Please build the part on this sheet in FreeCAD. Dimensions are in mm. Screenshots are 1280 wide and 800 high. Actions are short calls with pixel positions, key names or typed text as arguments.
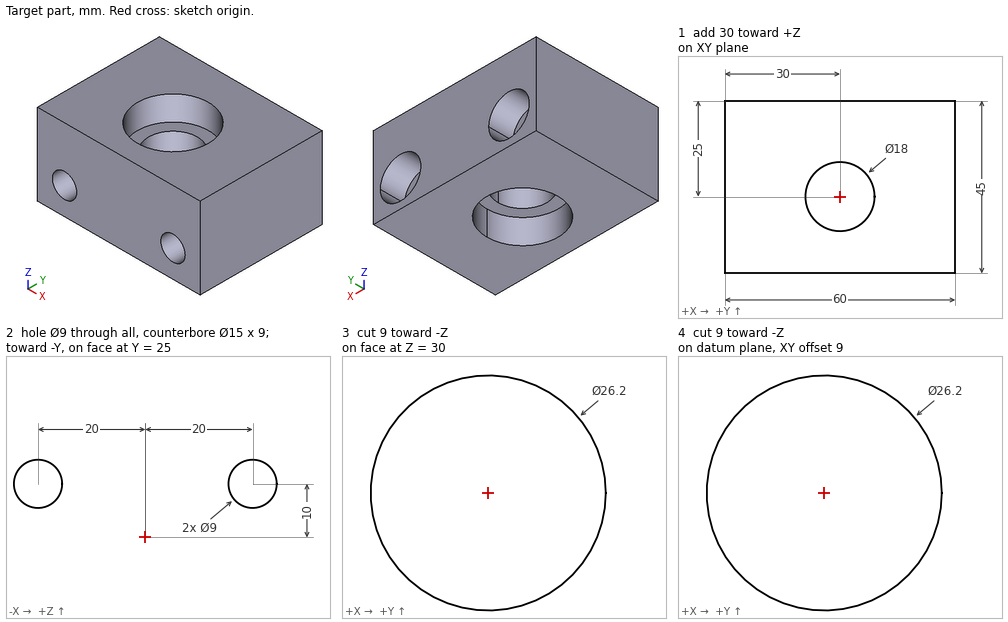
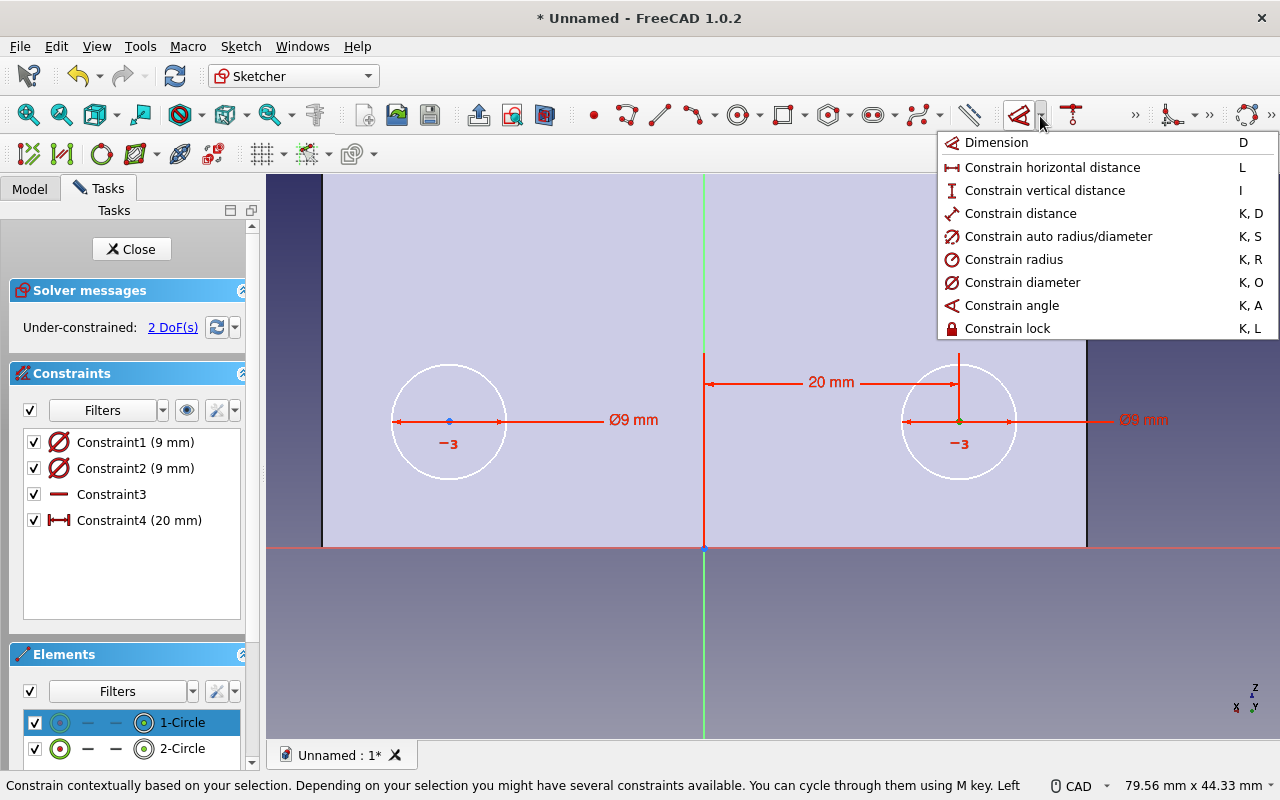
click(1108, 190)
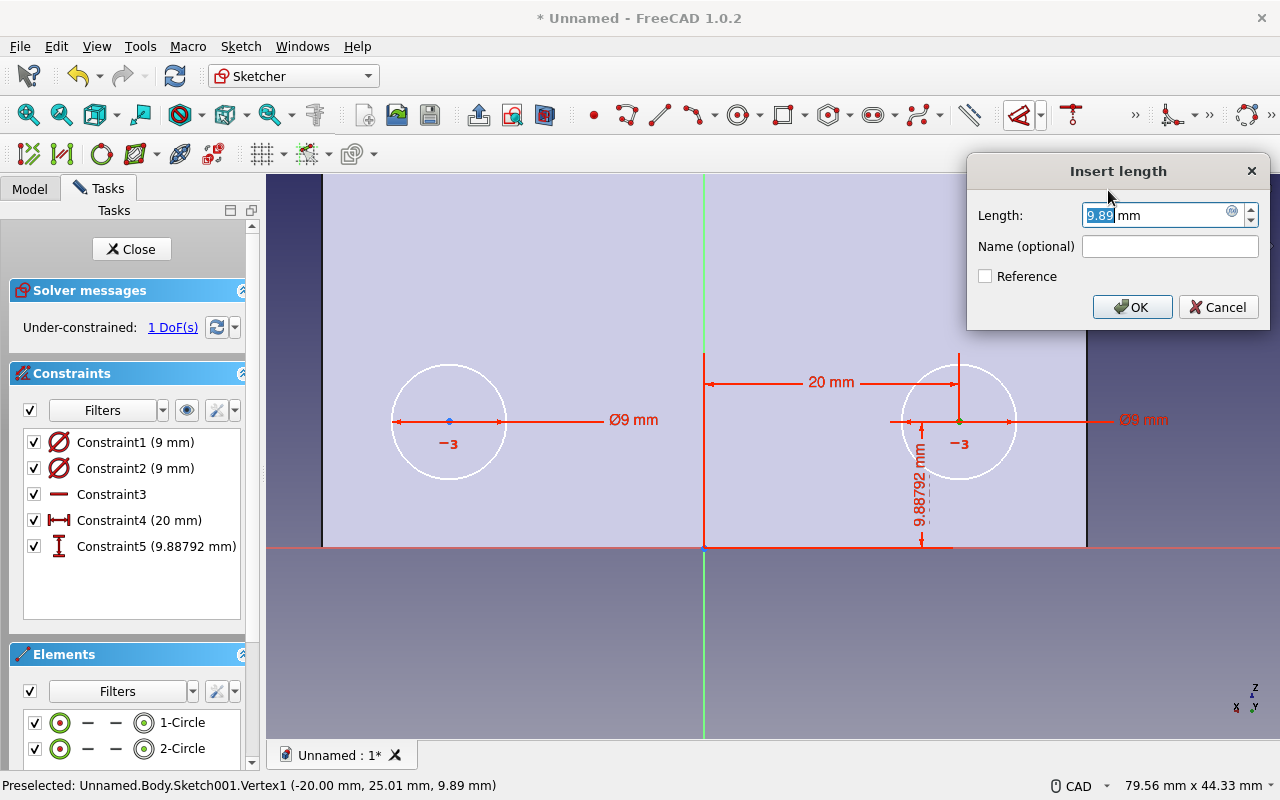
text(10)
key(Return)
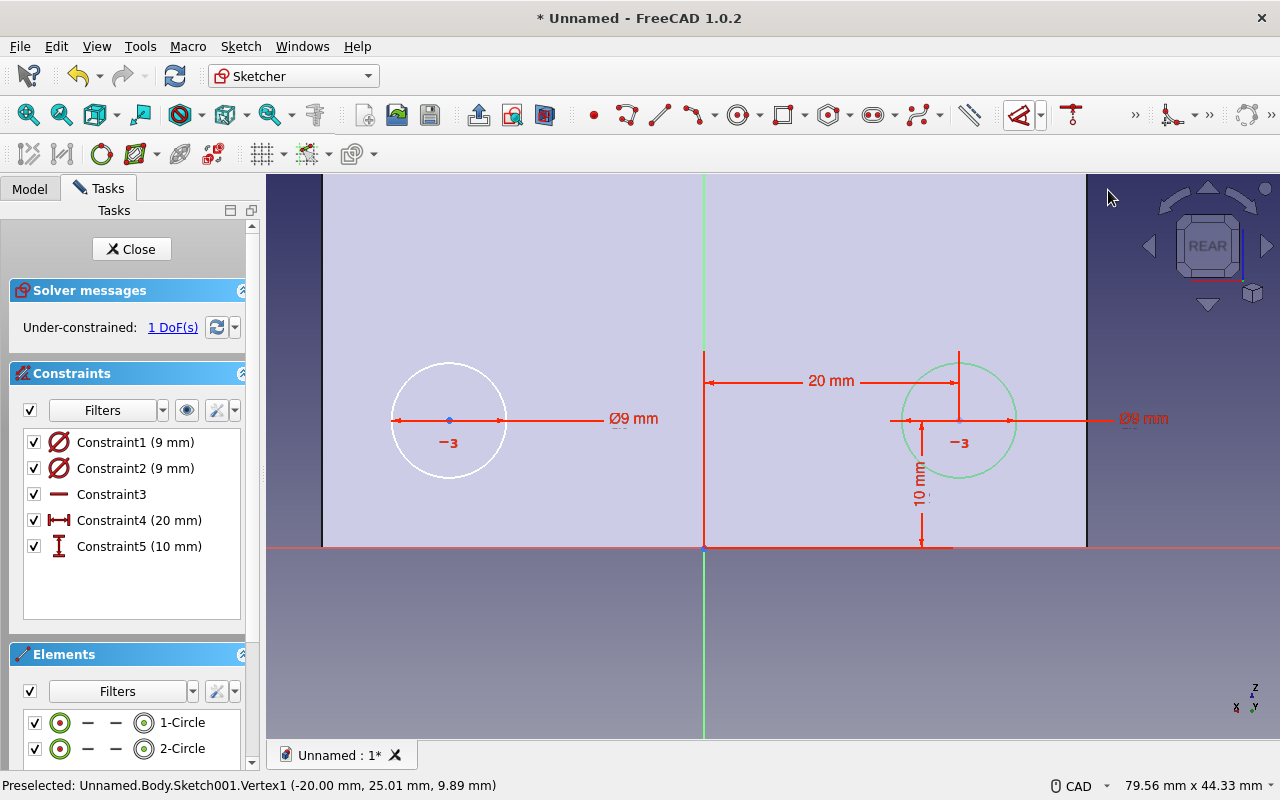
click(449, 421)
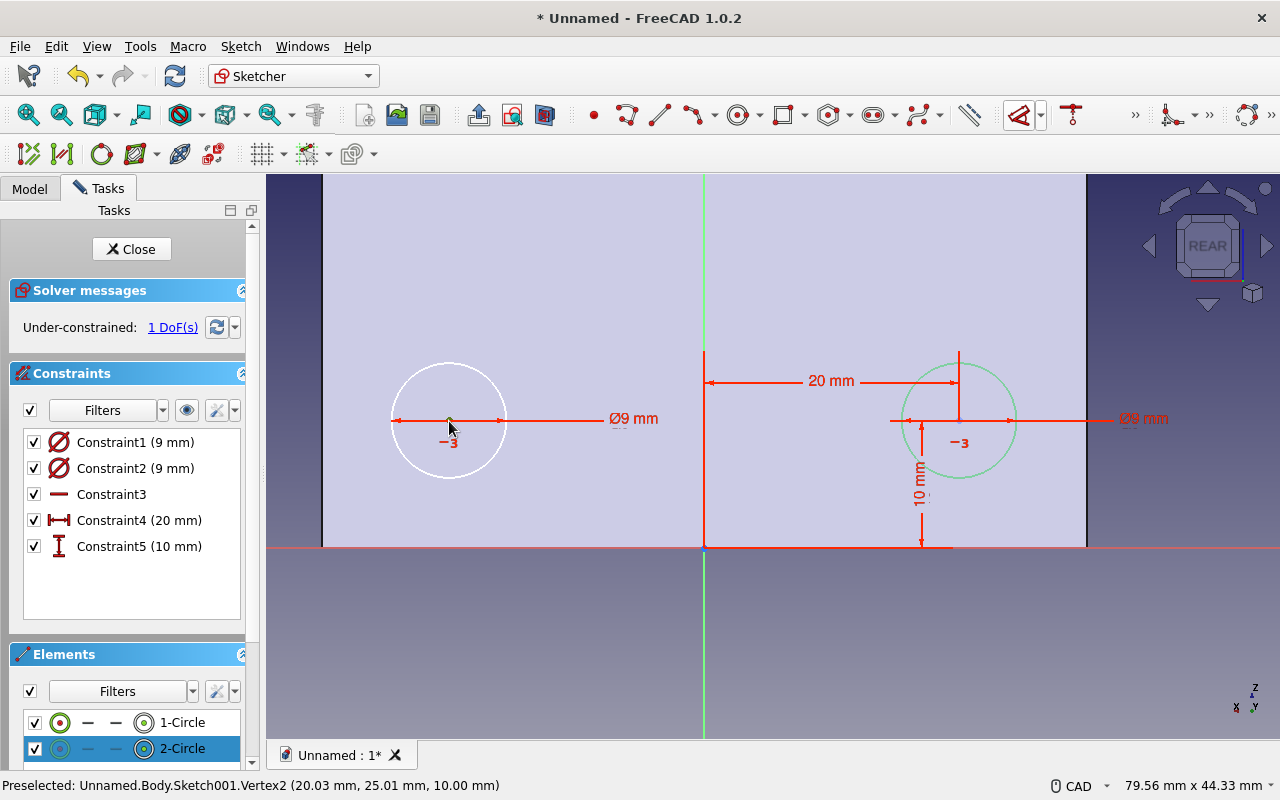
key(l)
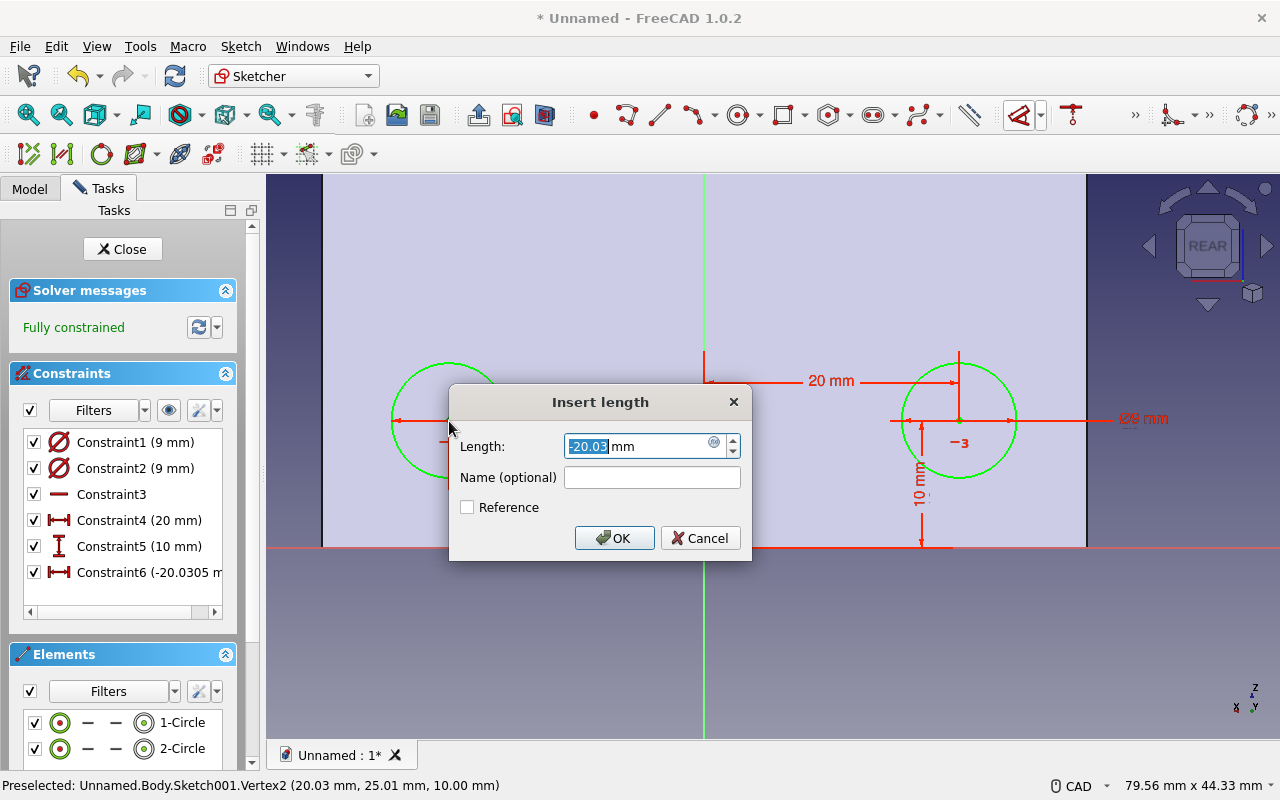
text(-20)
key(Return)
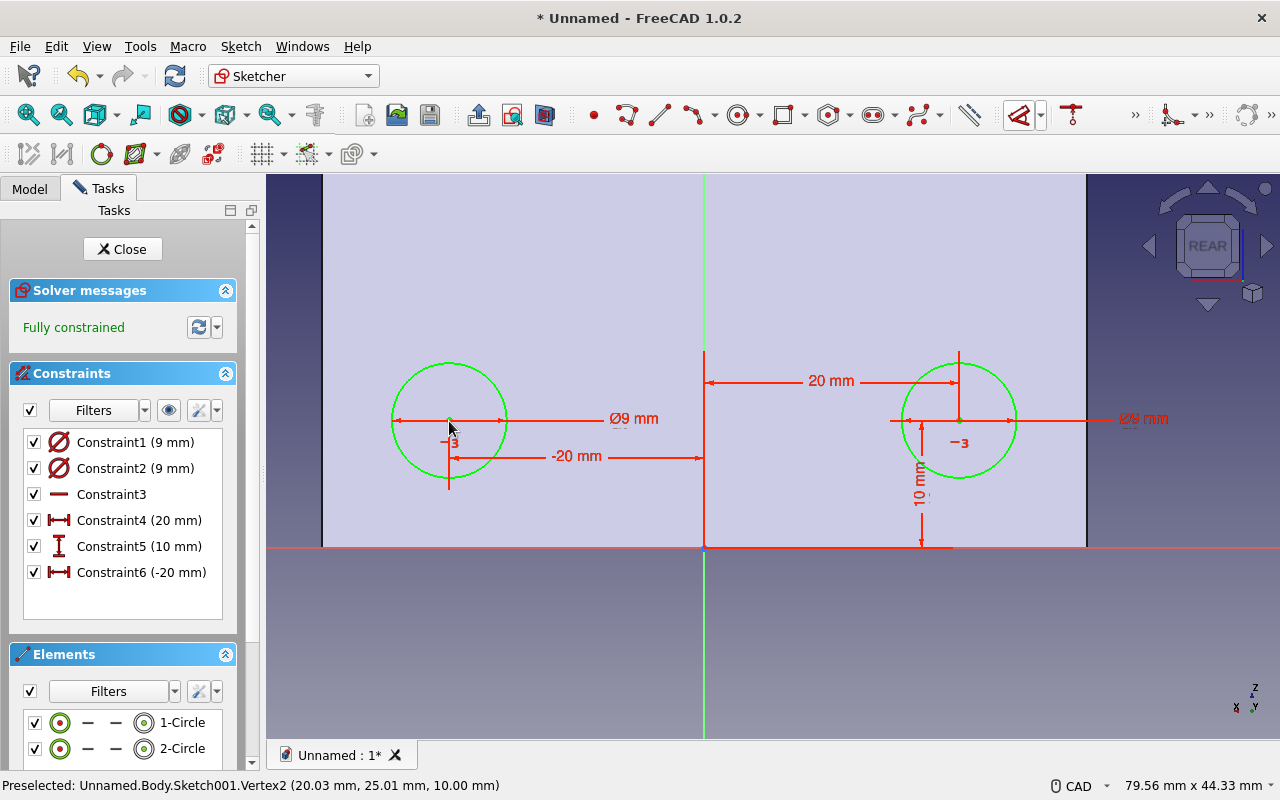
click(123, 249)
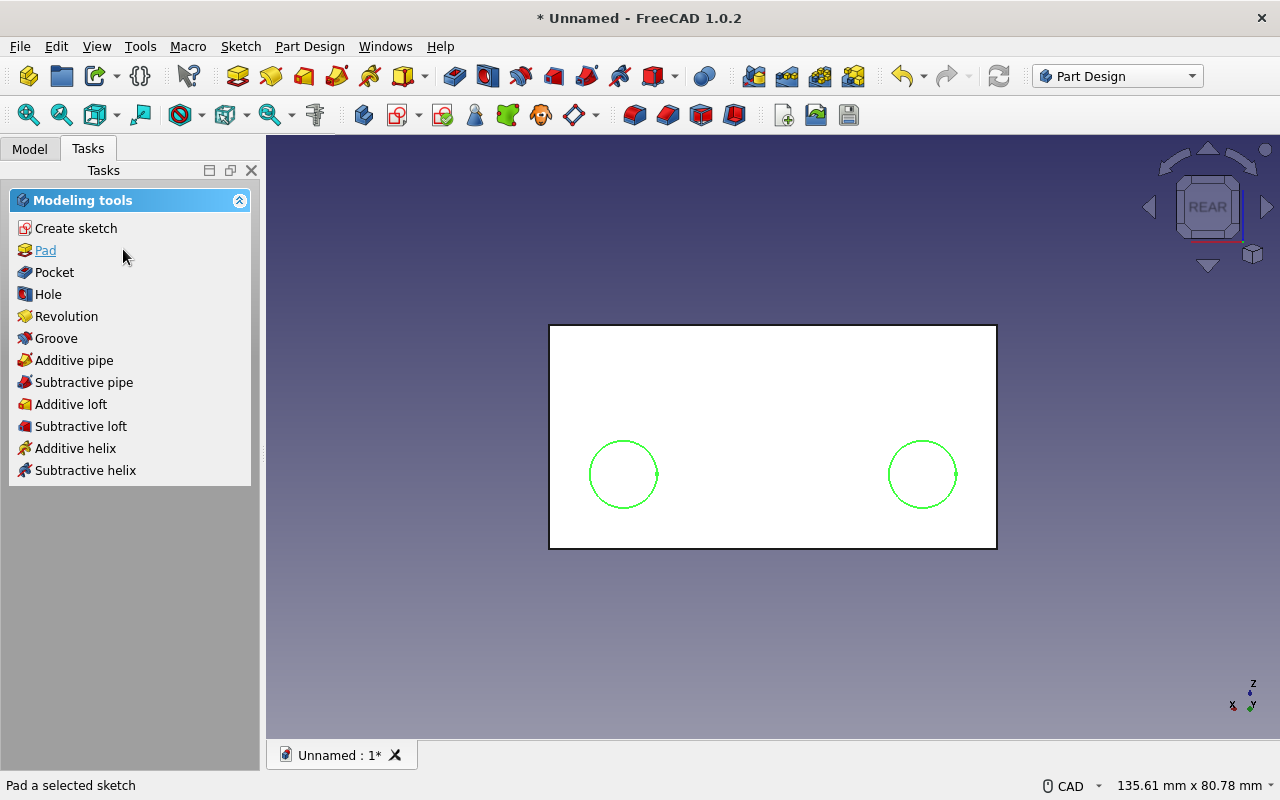
click(488, 76)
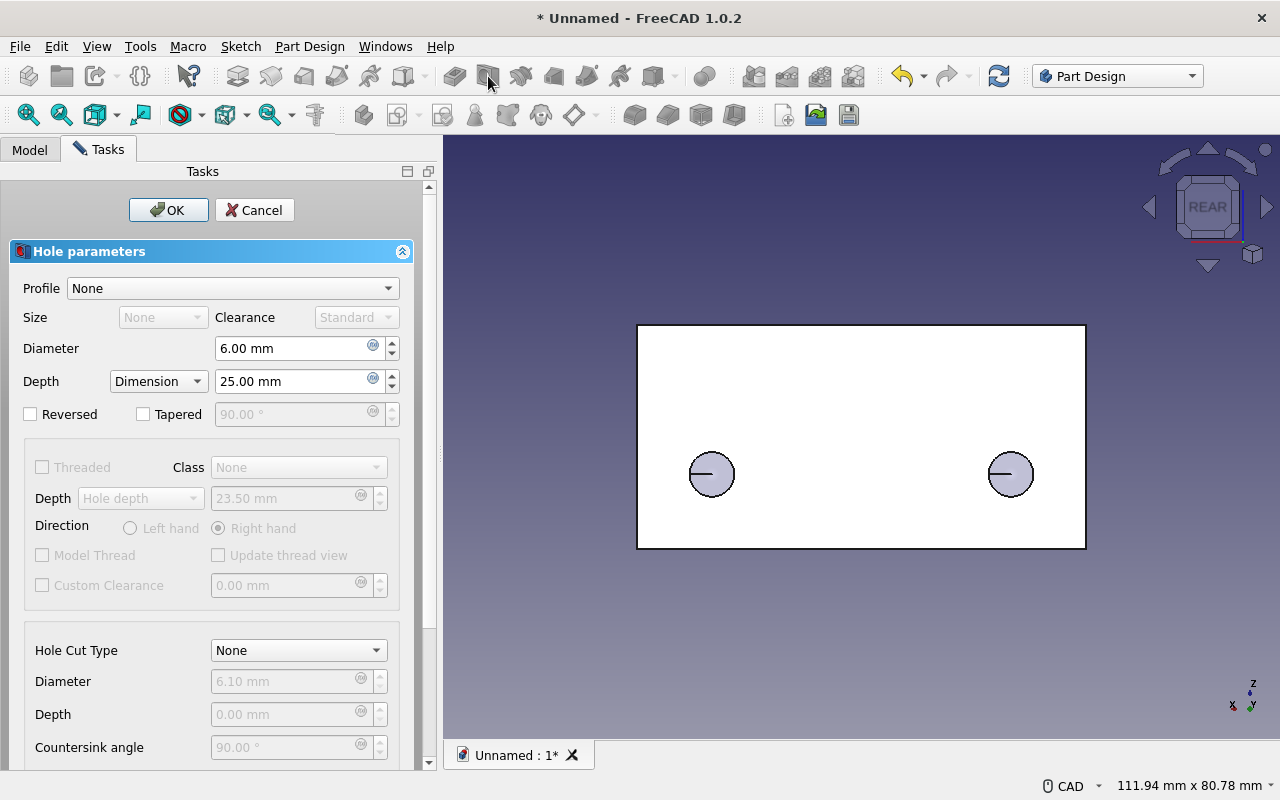
triple_click(300, 348)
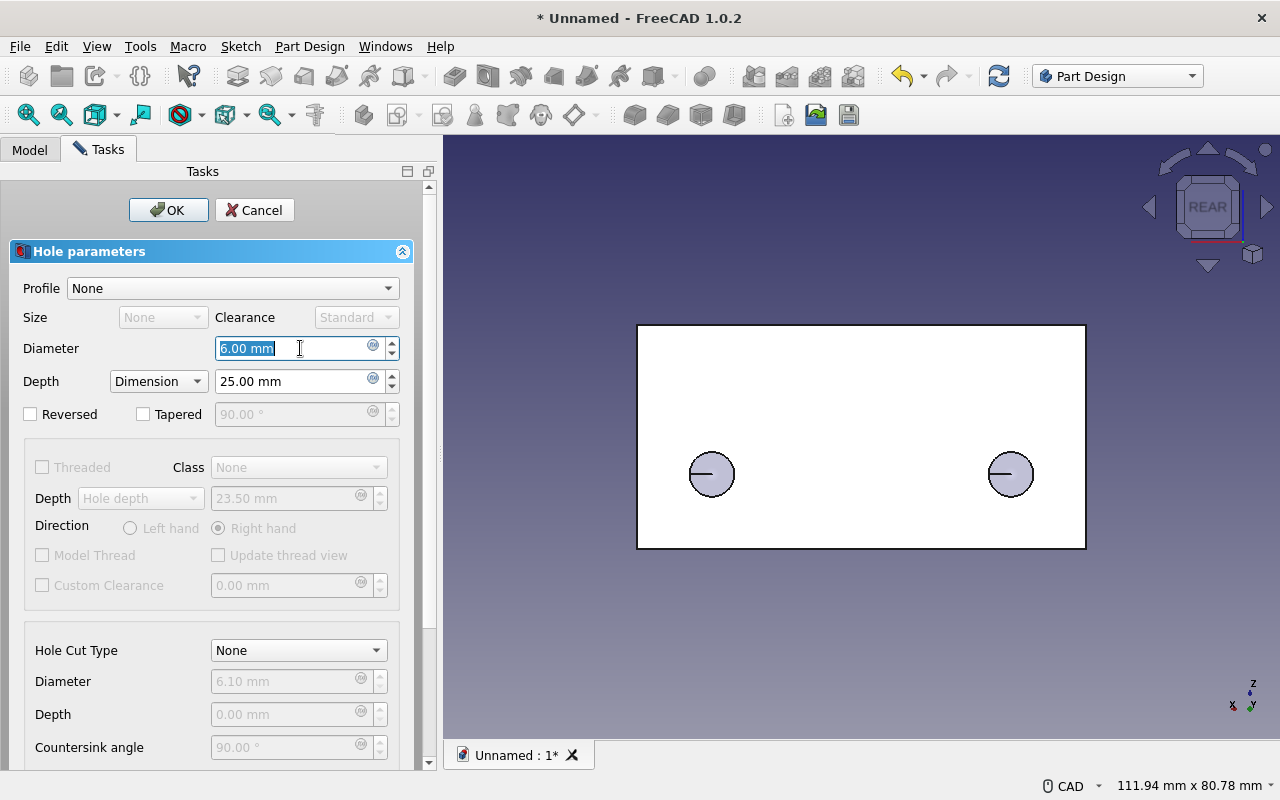
text(9)
key(Tab)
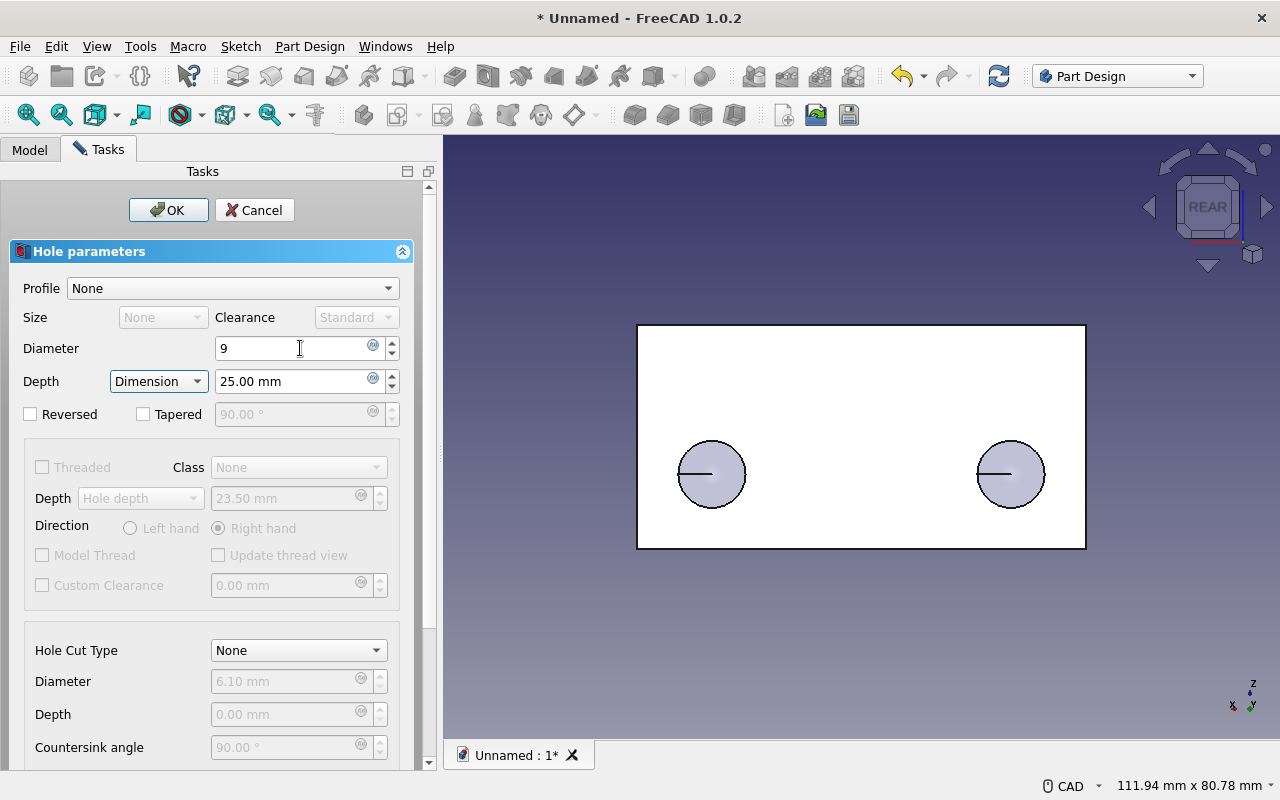
click(160, 382)